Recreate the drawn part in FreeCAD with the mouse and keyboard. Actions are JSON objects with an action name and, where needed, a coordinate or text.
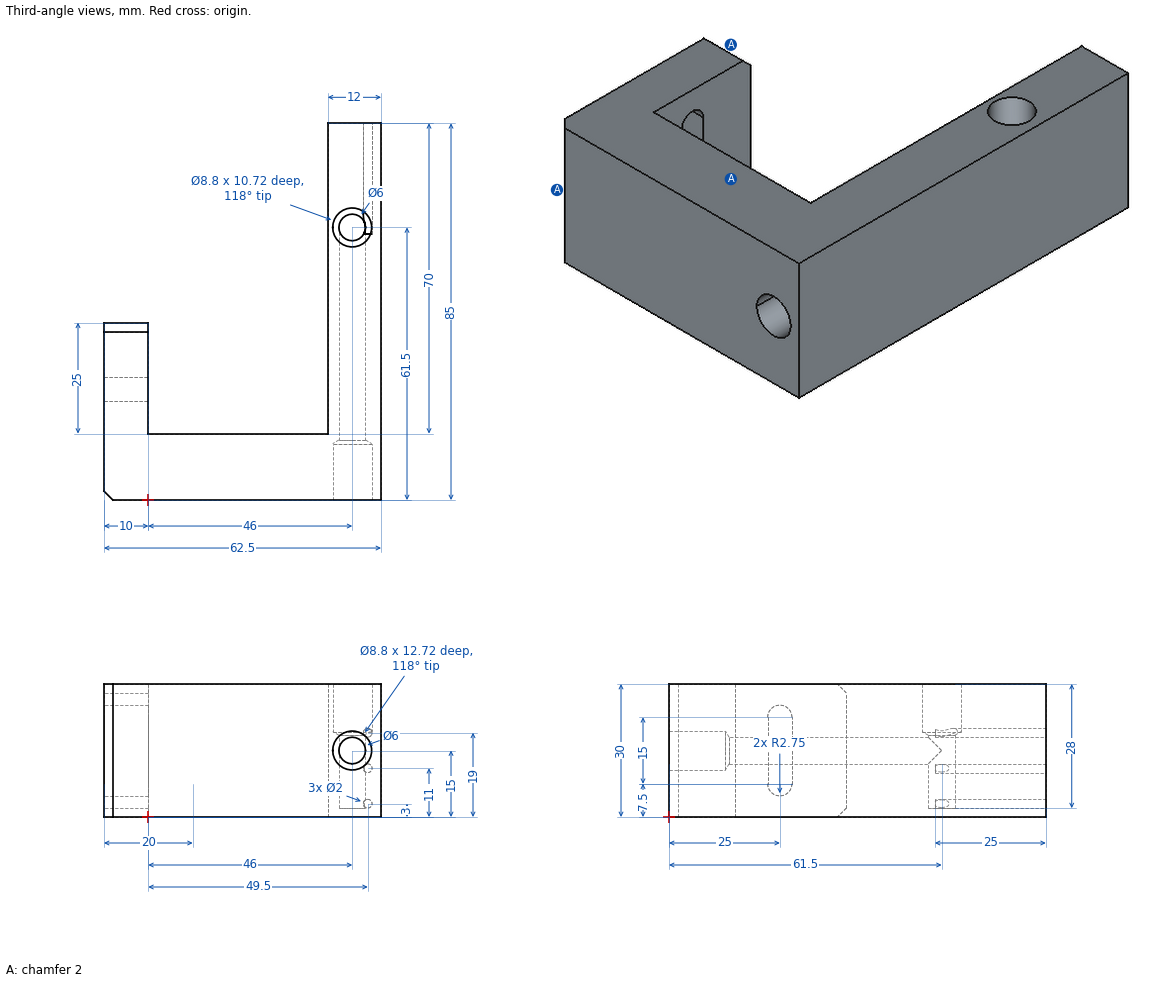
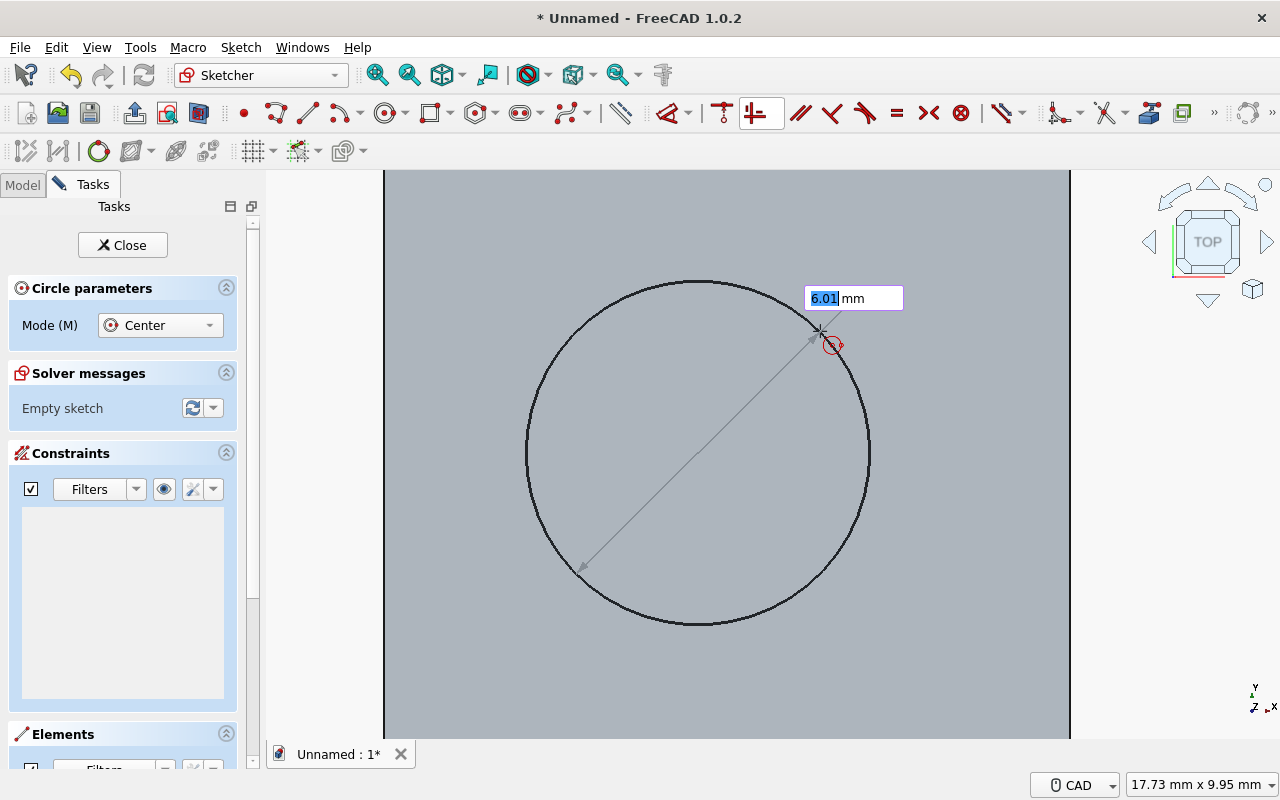
{"action": "type", "text": "6"}
{"action": "key", "text": "Return"}
{"action": "key", "text": "Escape"}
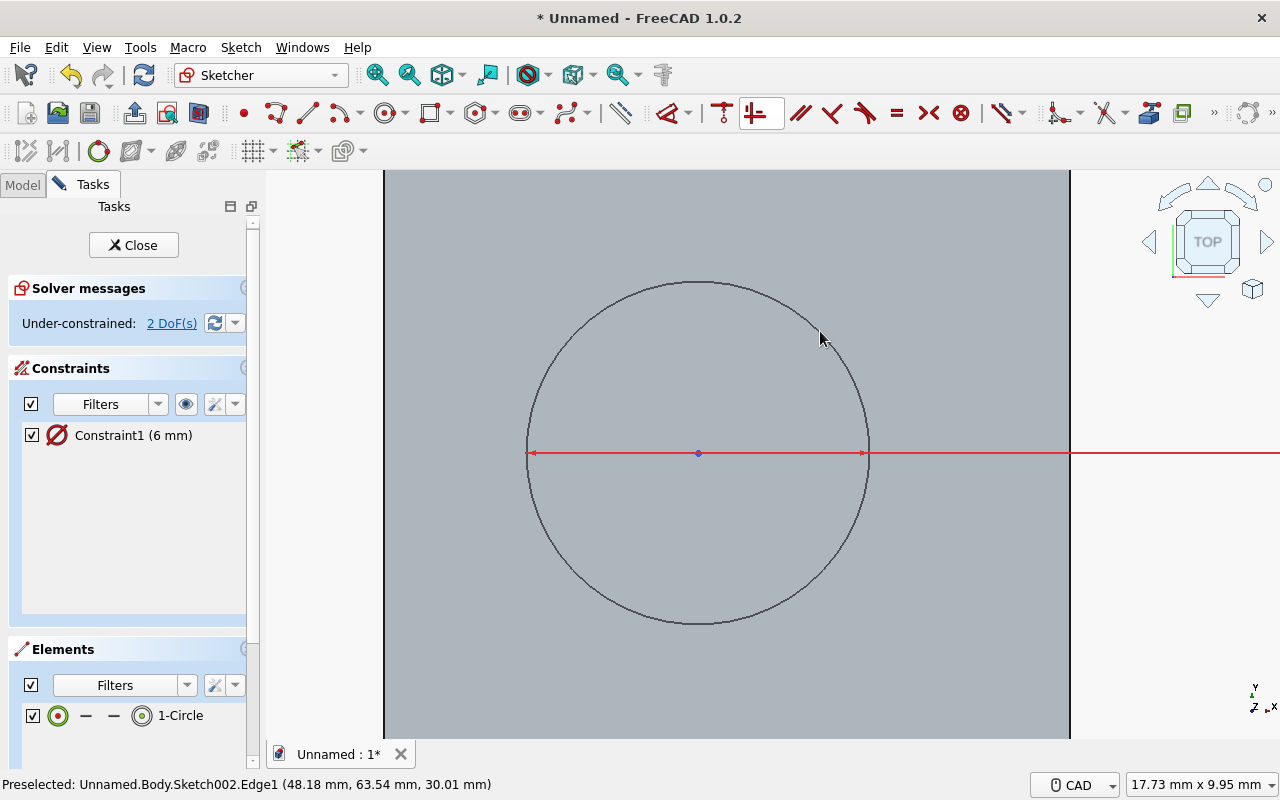
{"action": "key", "text": "d"}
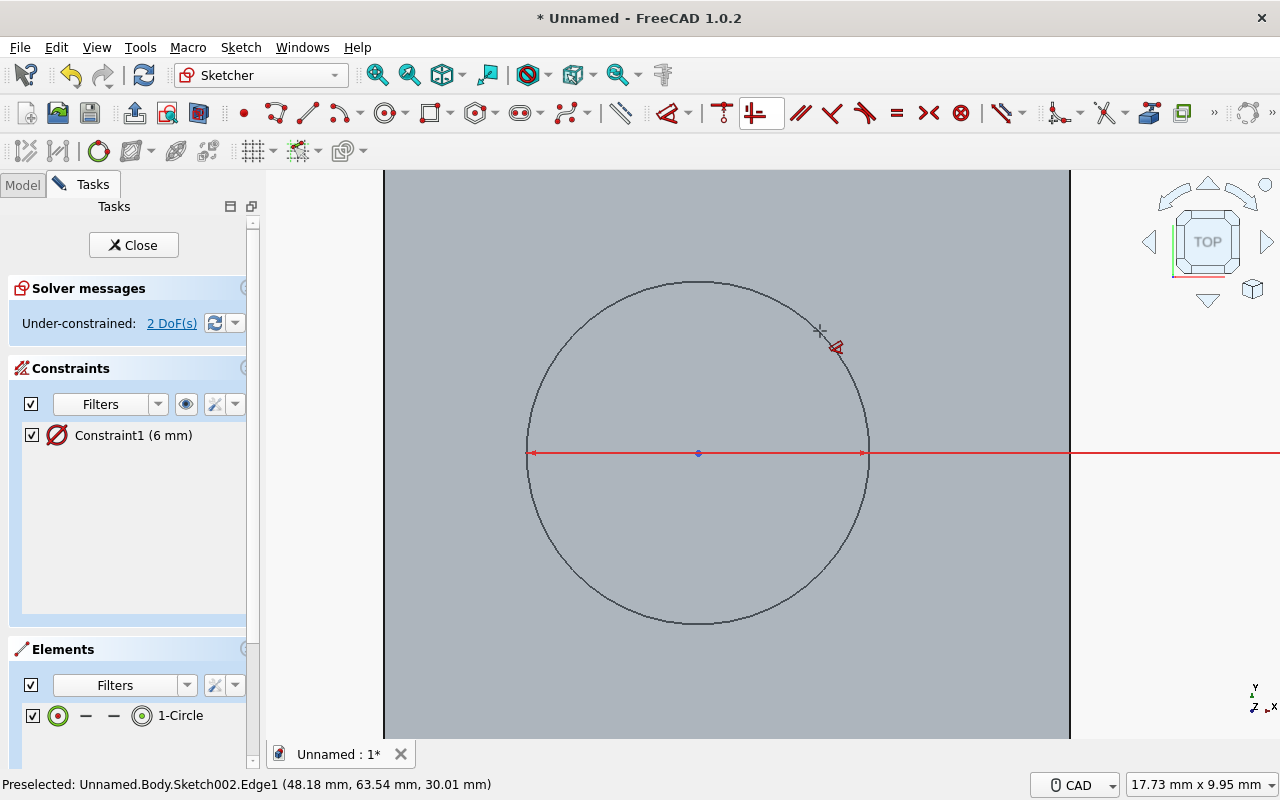
{"action": "left_click", "coordinate": [698, 453]}
{"action": "left_click", "coordinate": [496, 419]}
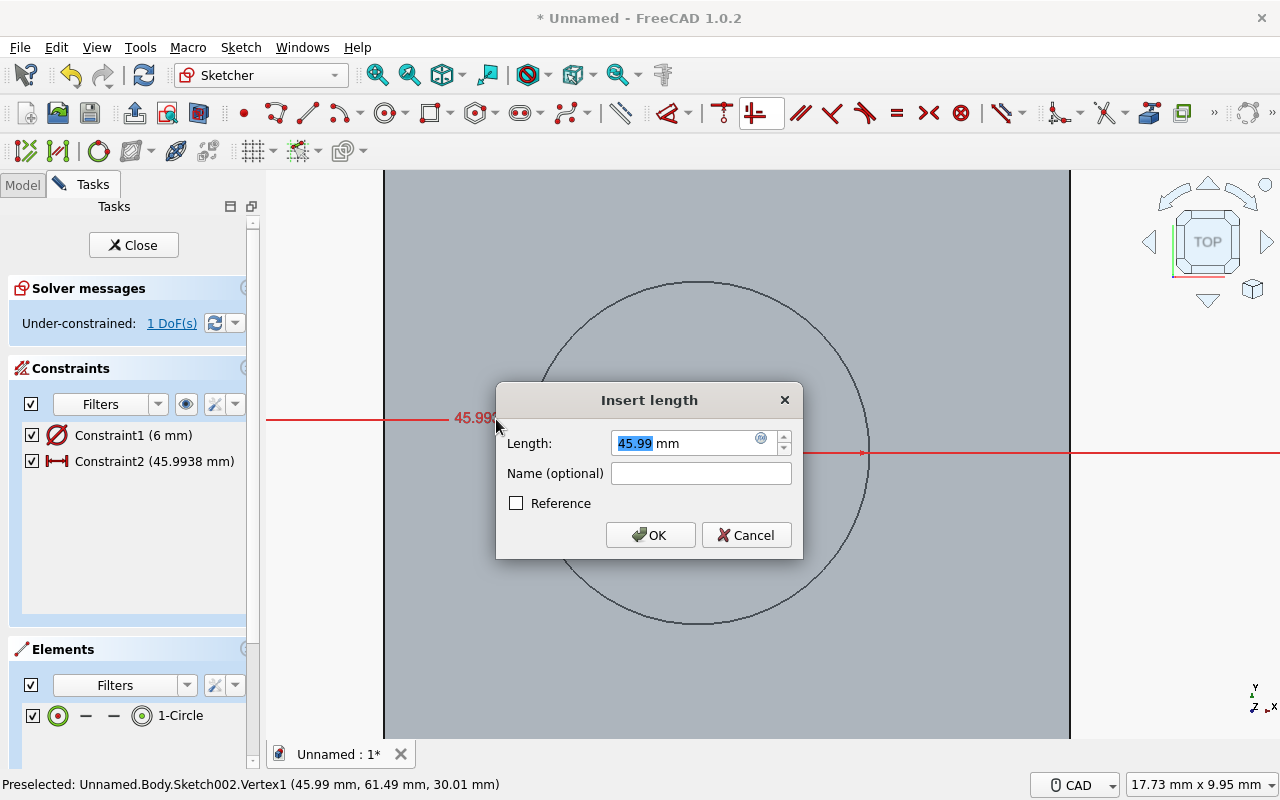
{"action": "type", "text": "46"}
{"action": "key", "text": "Return"}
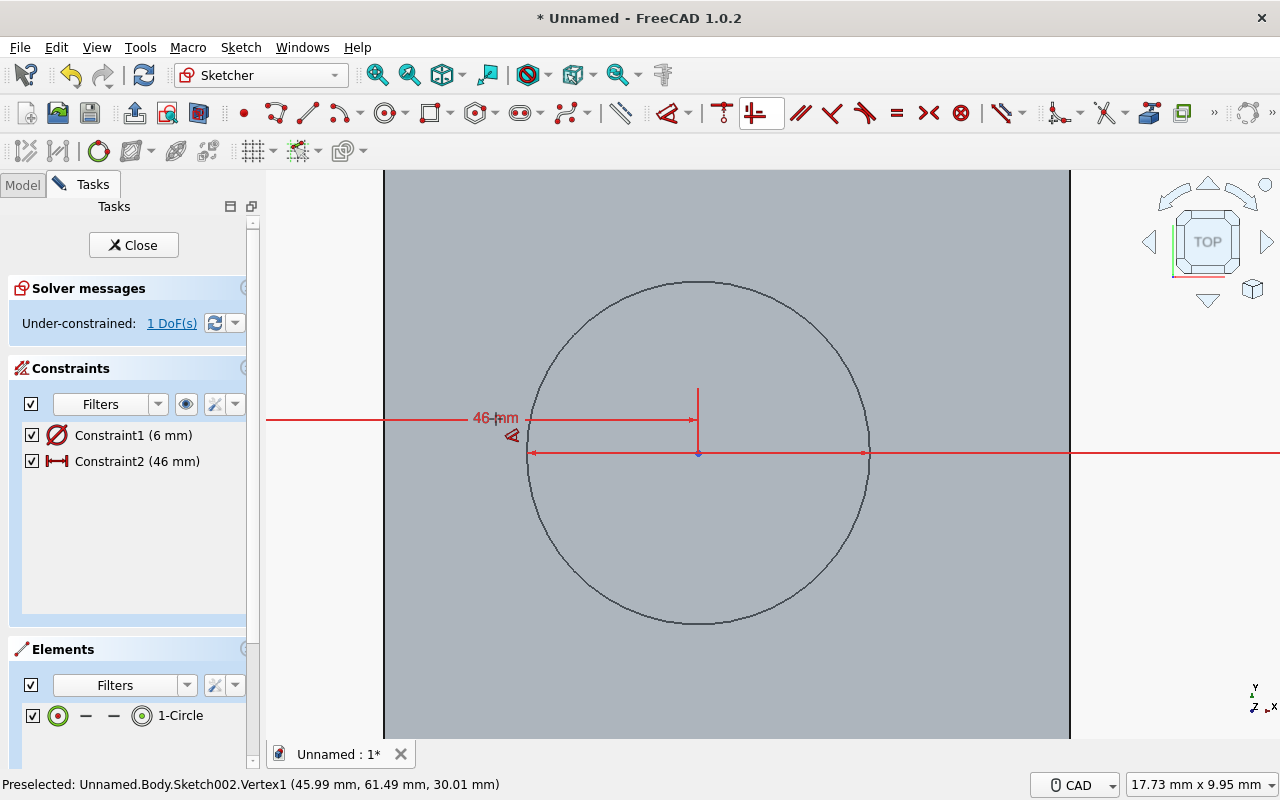
{"action": "left_click", "coordinate": [698, 453]}
{"action": "left_click", "coordinate": [732, 582]}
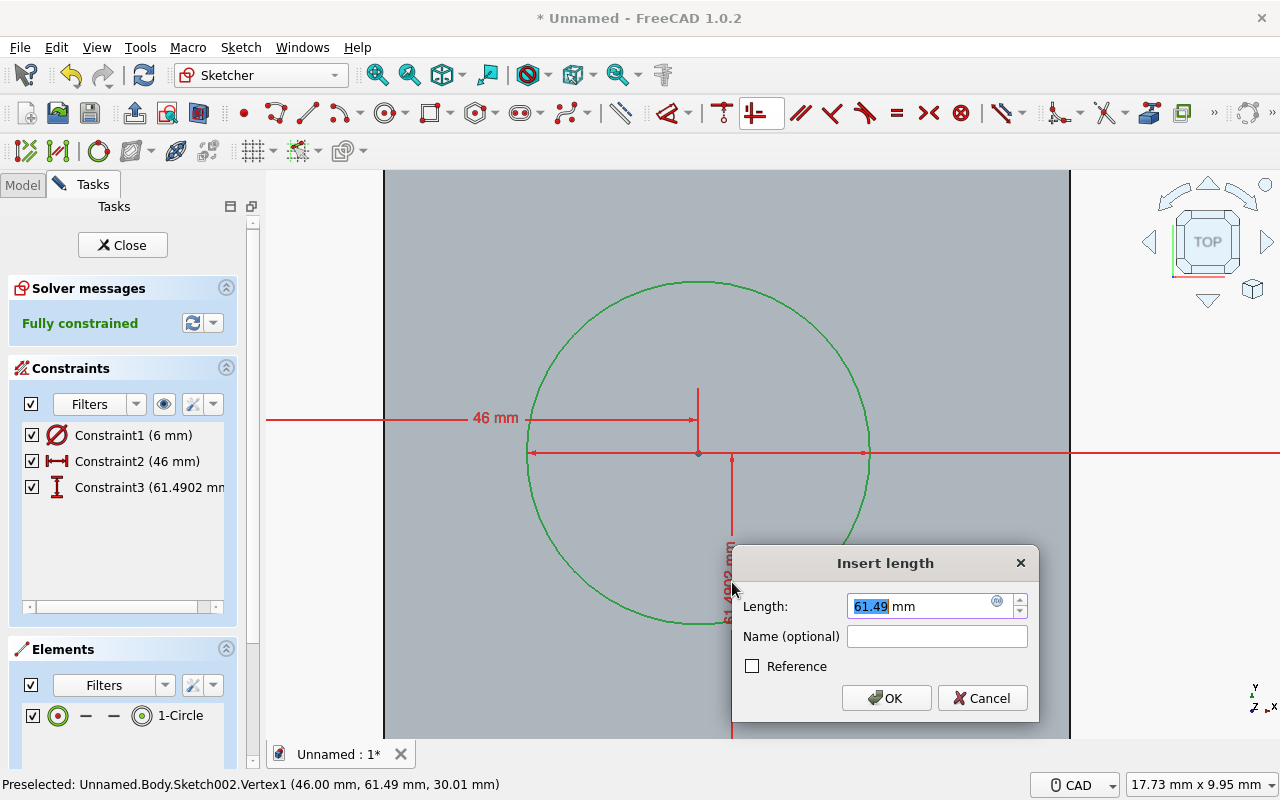
{"action": "type", "text": "61.5"}
{"action": "key", "text": "Return"}
{"action": "key", "text": "Escape"}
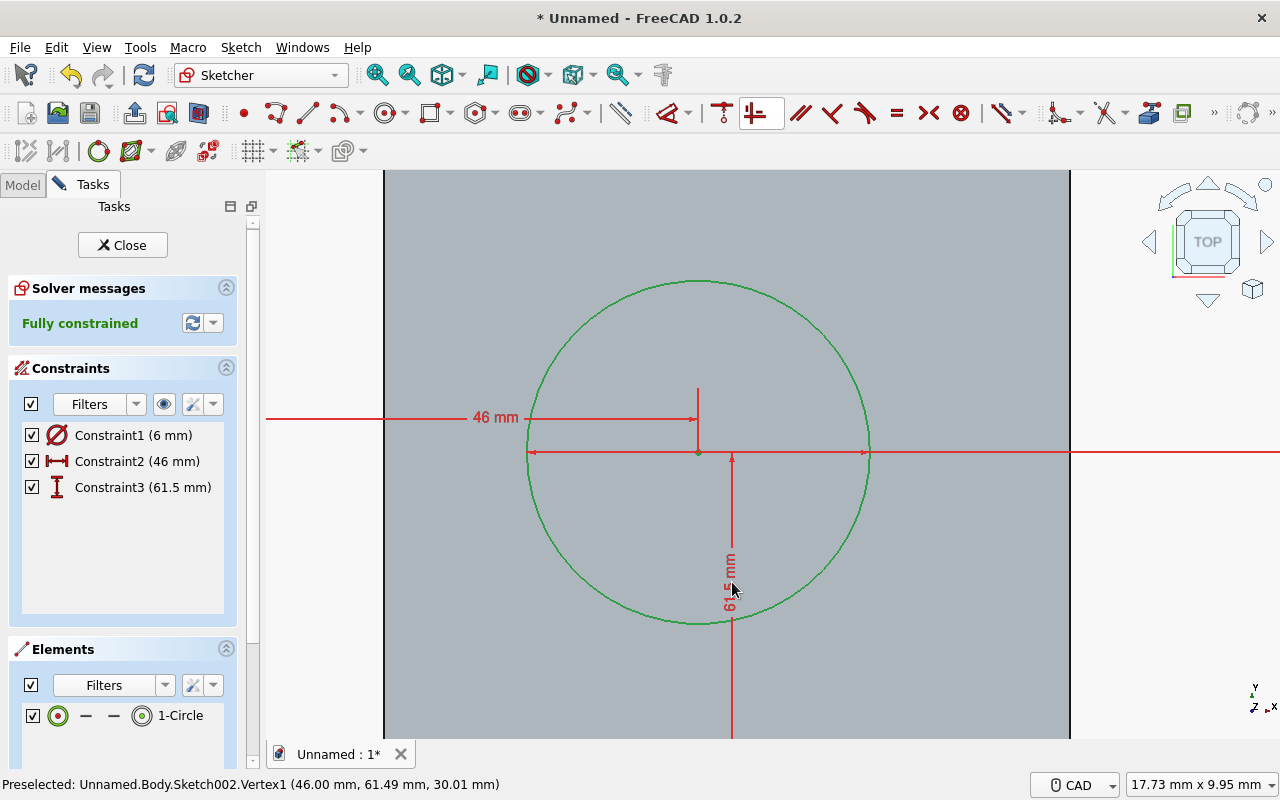
{"action": "left_click", "coordinate": [123, 245]}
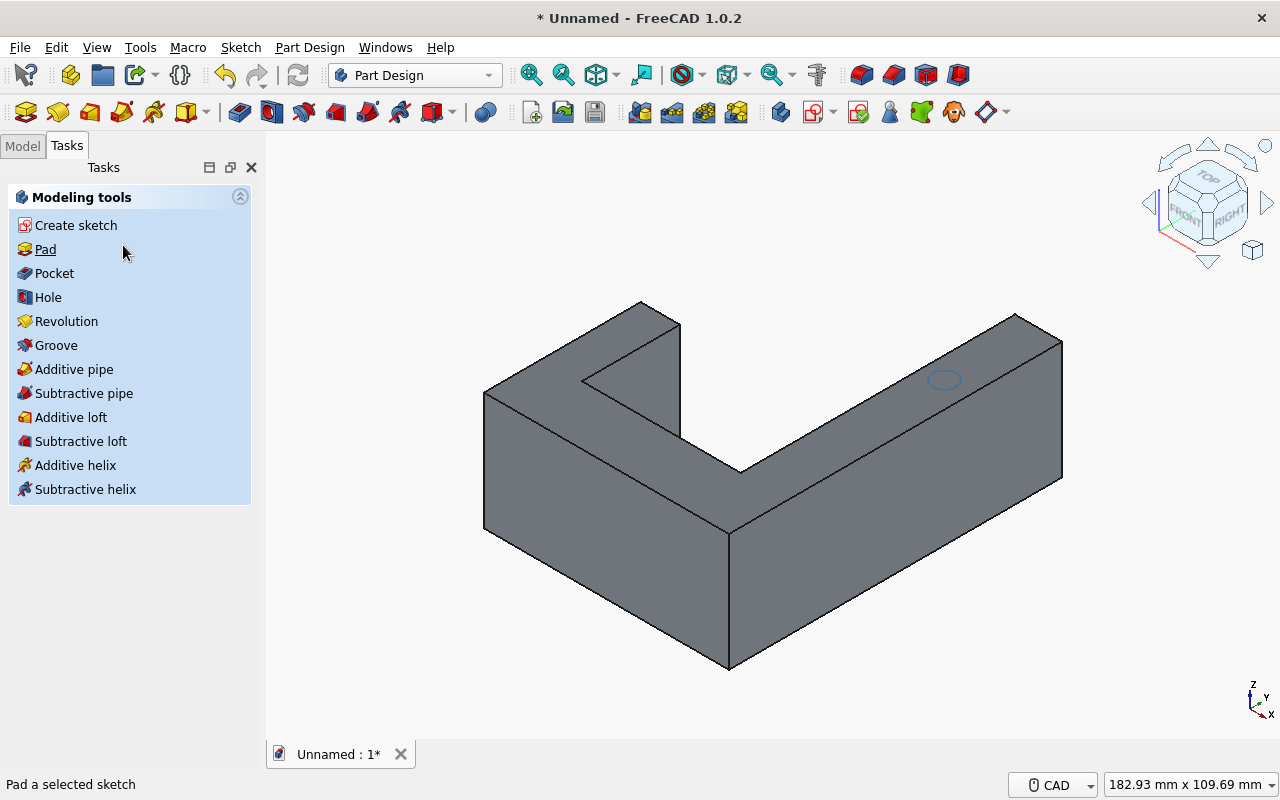
{"action": "left_click", "coordinate": [240, 112]}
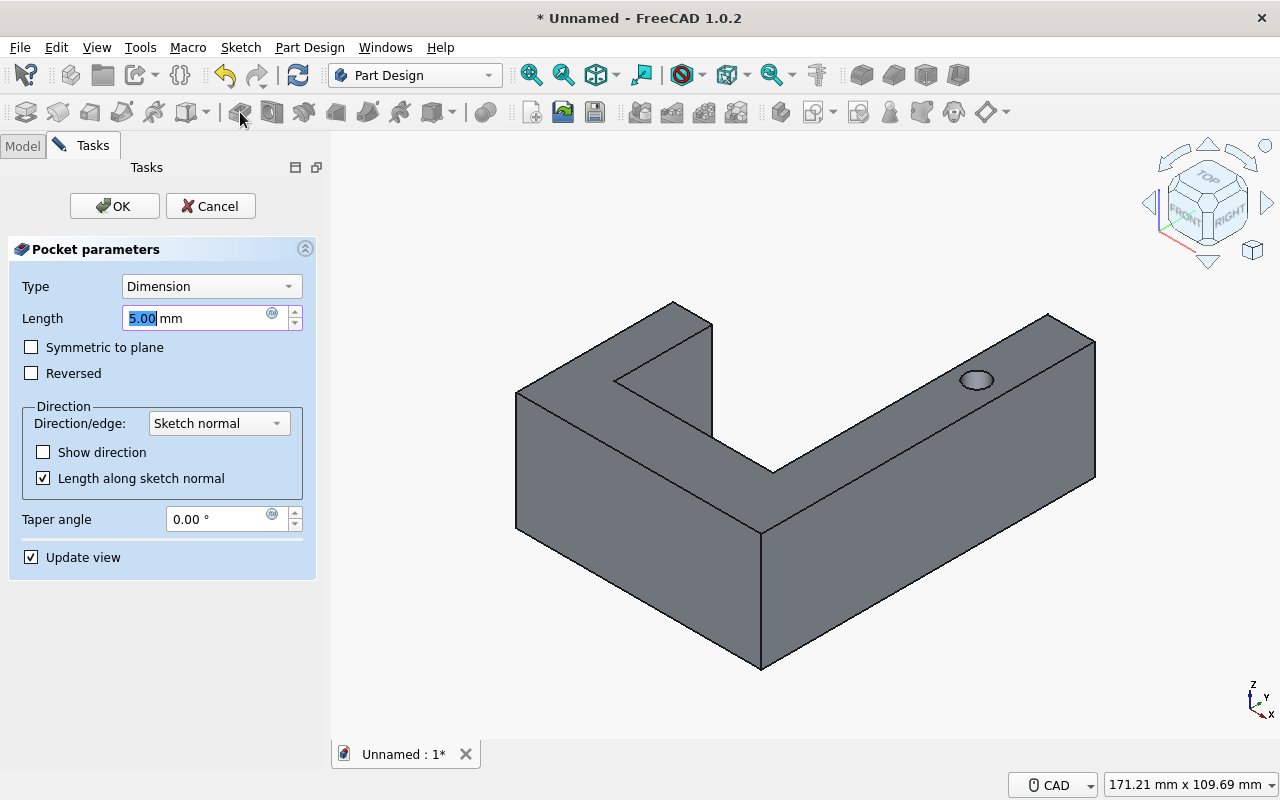
{"action": "type", "text": "28"}
{"action": "key", "text": "Tab"}